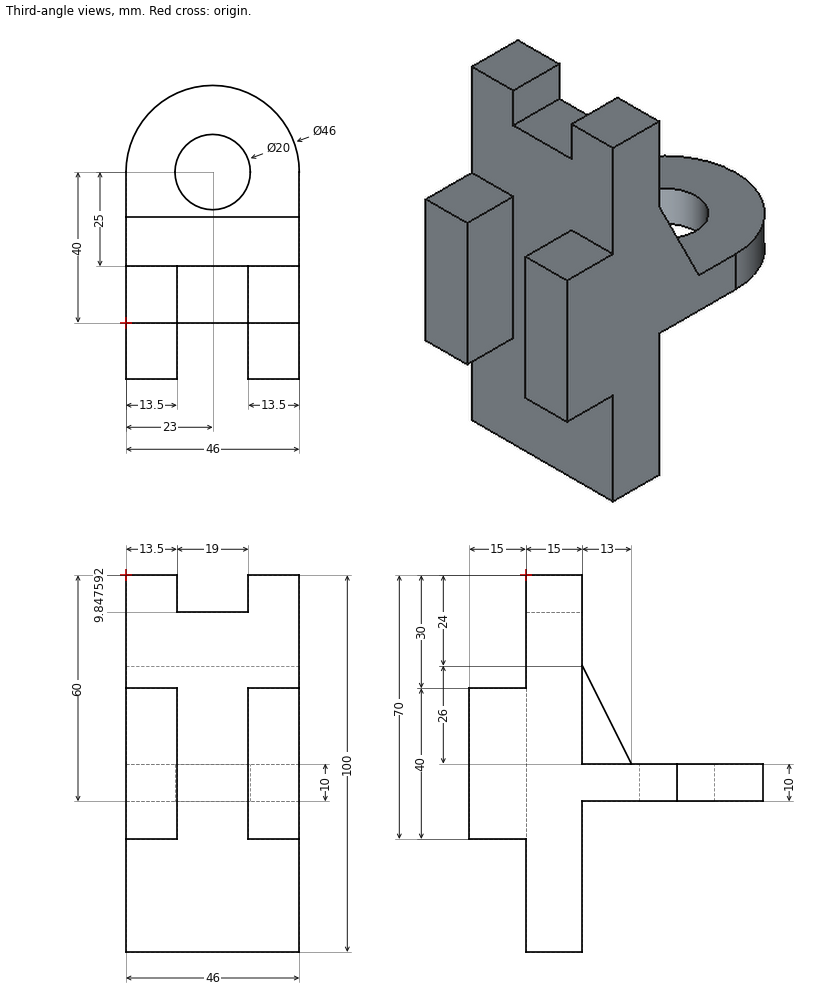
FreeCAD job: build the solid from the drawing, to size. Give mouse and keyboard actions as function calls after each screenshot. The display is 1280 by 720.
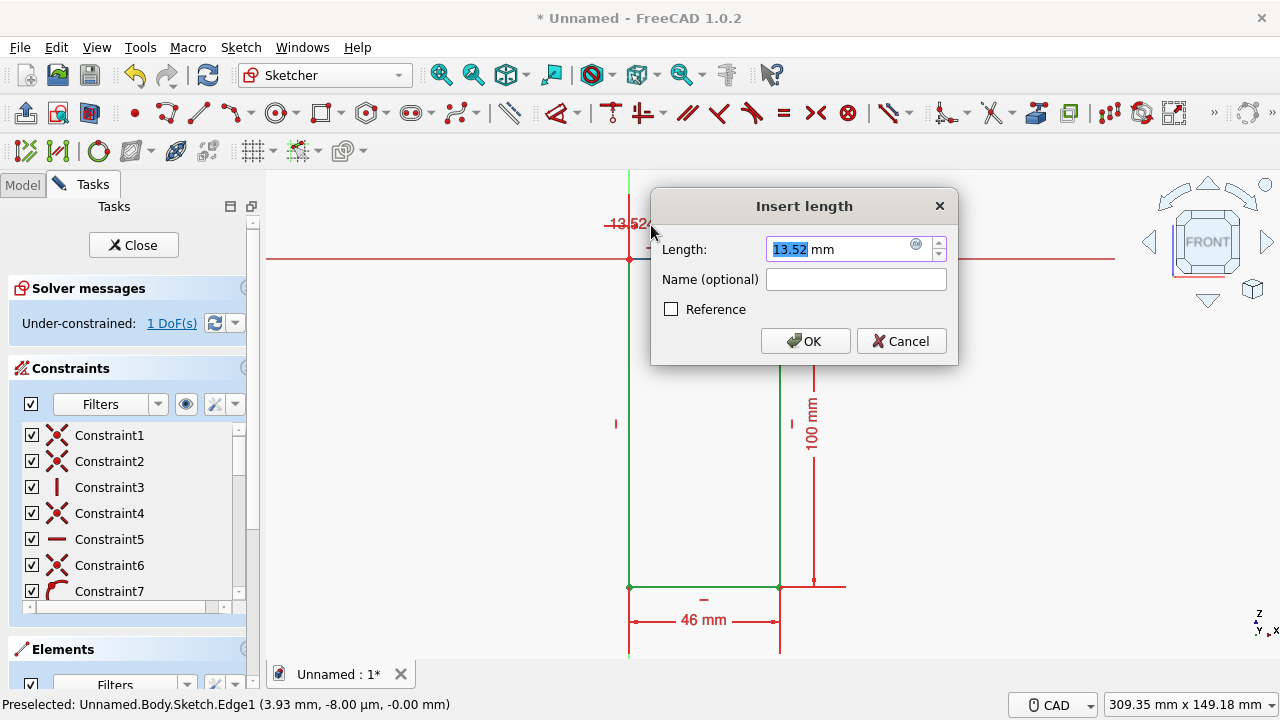
text(13.5)
key(Return)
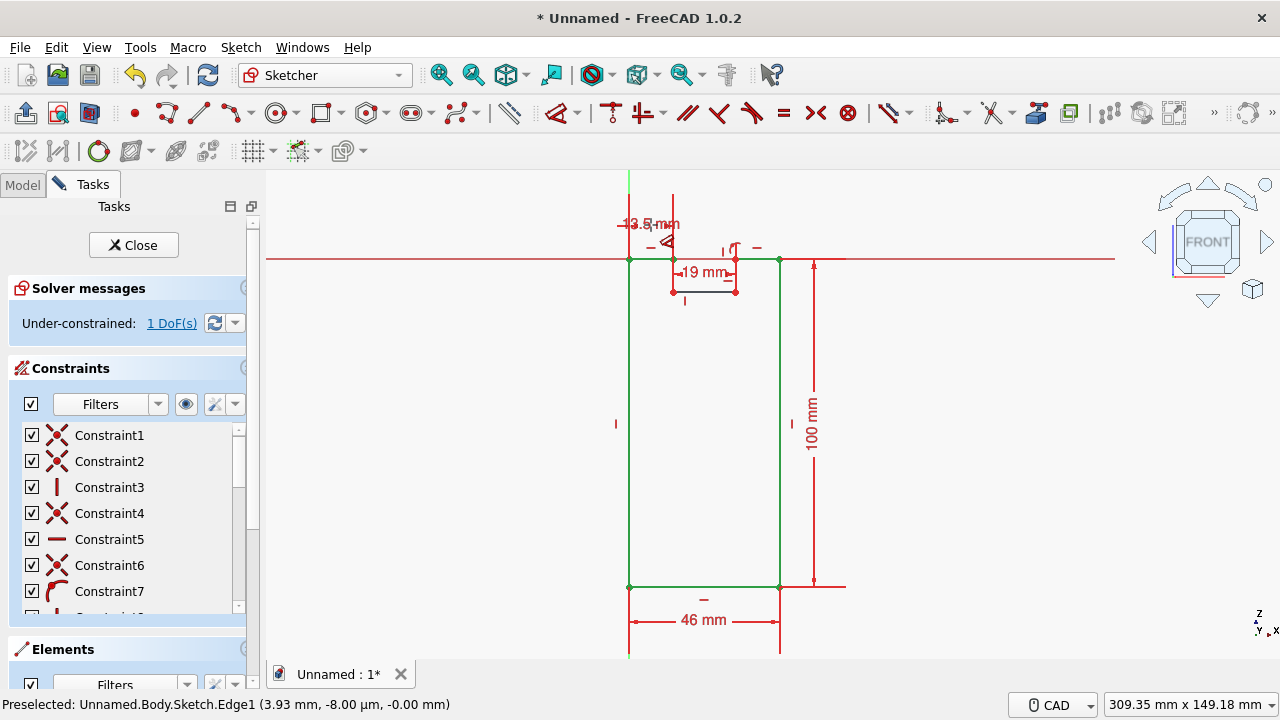
scroll(673, 269, up, 2)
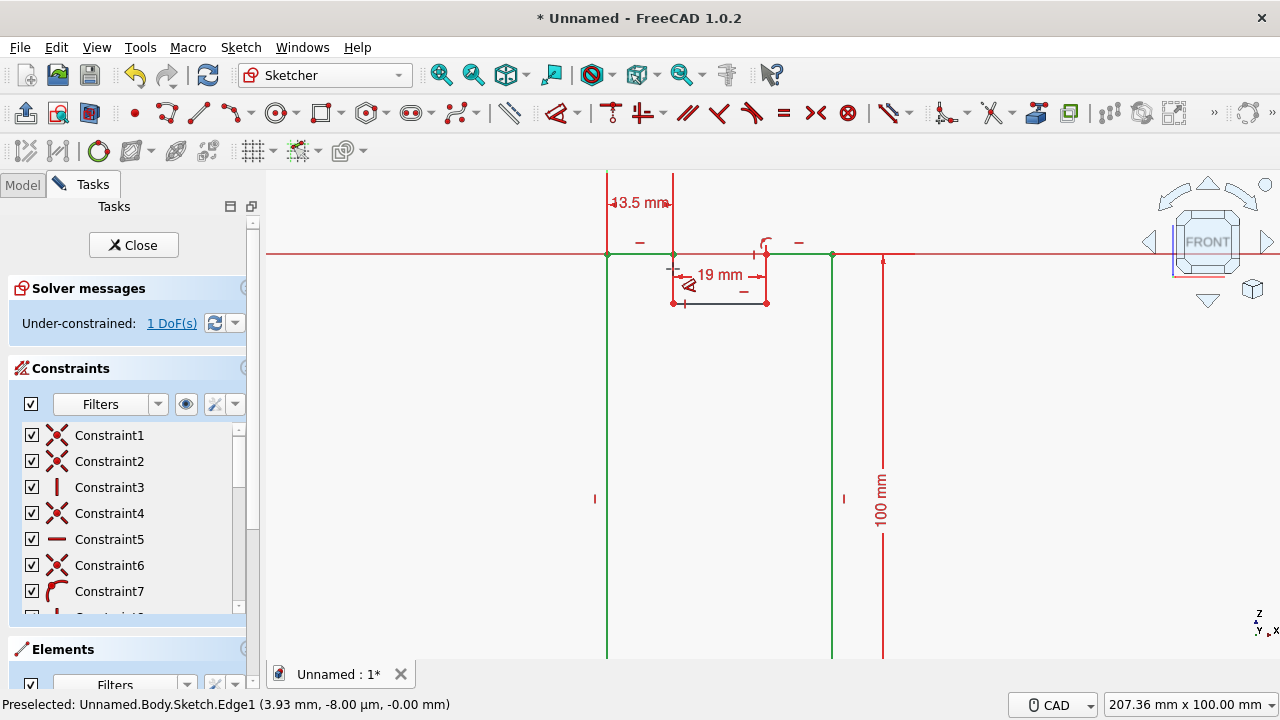
click(673, 269)
click(639, 279)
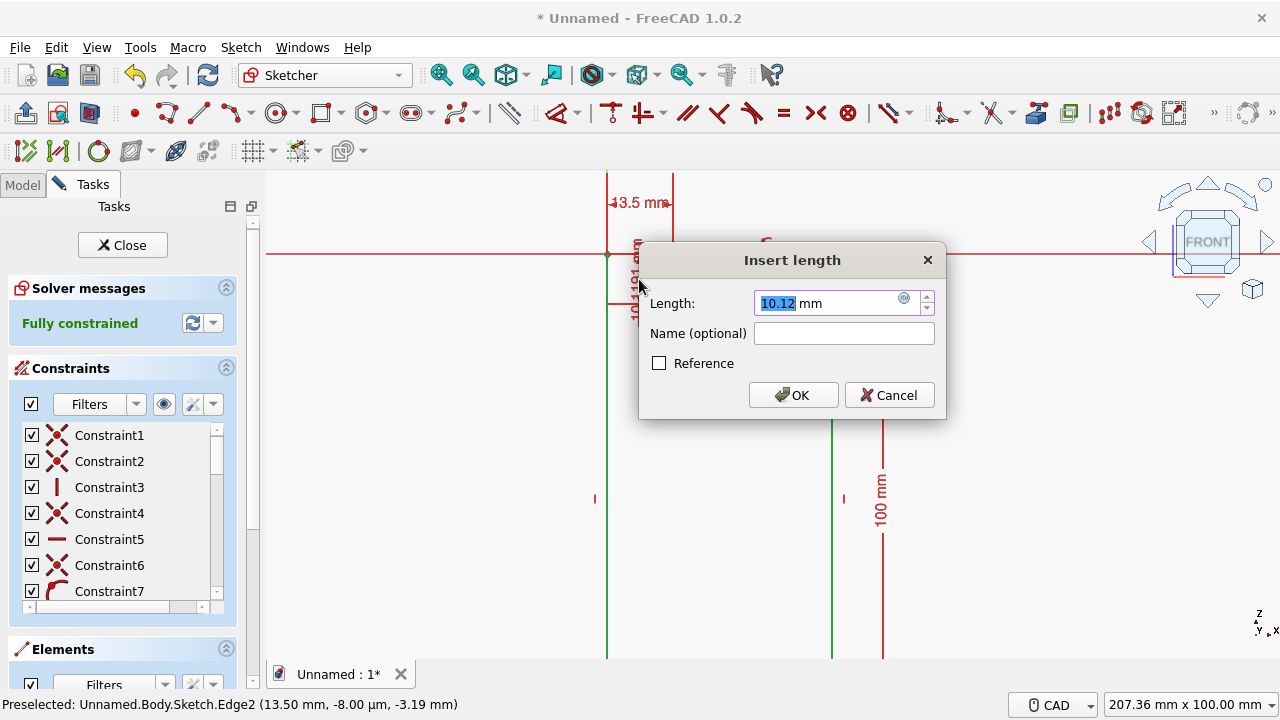
text(9.847592)
key(Return)
key(Escape)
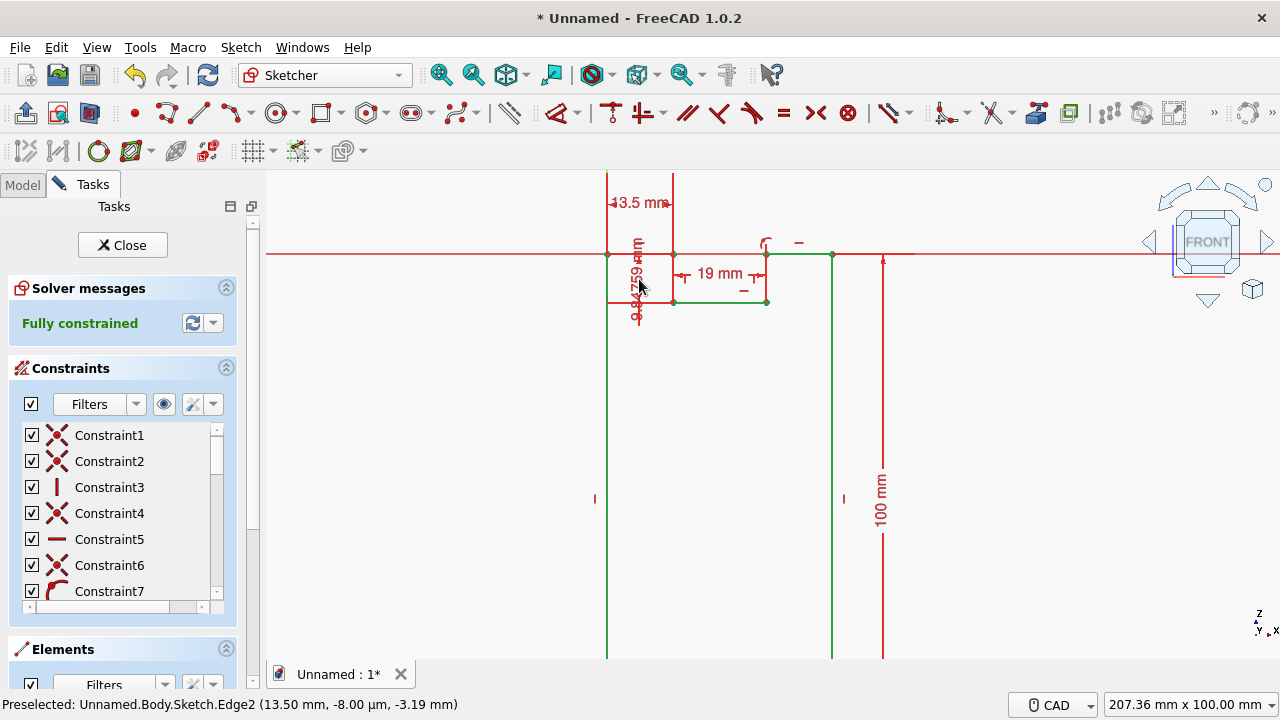
click(123, 245)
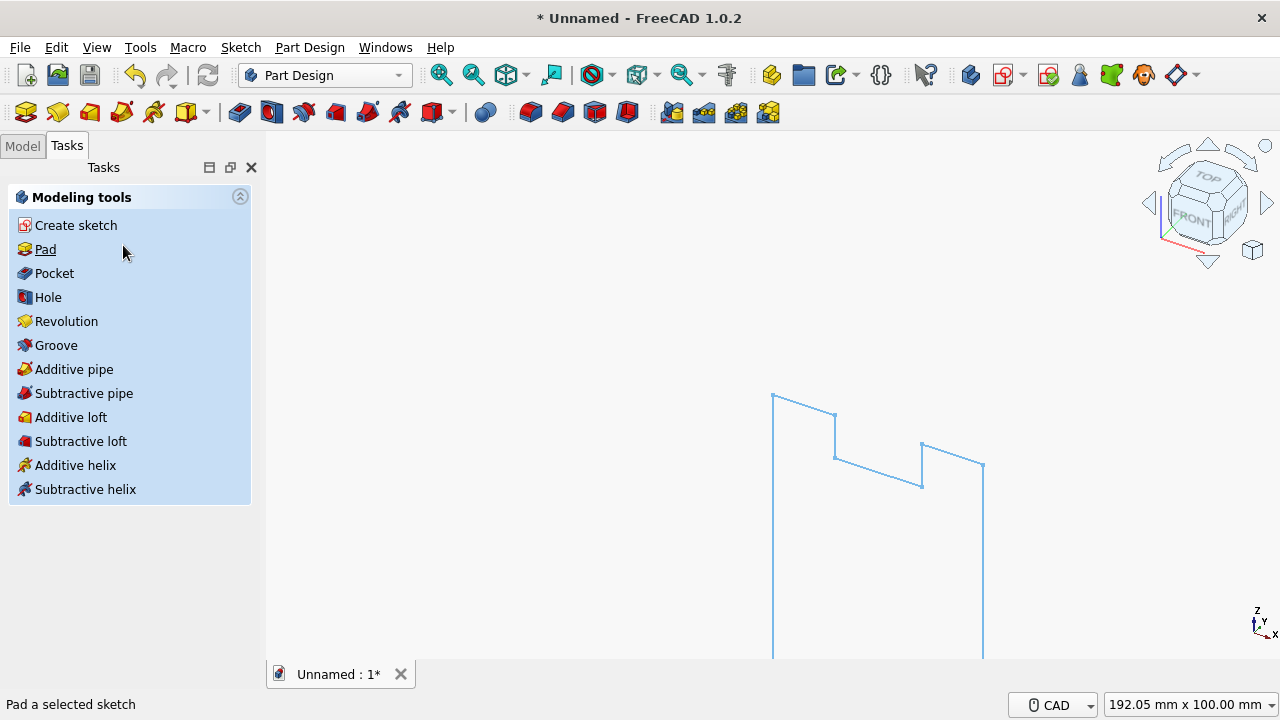
click(26, 112)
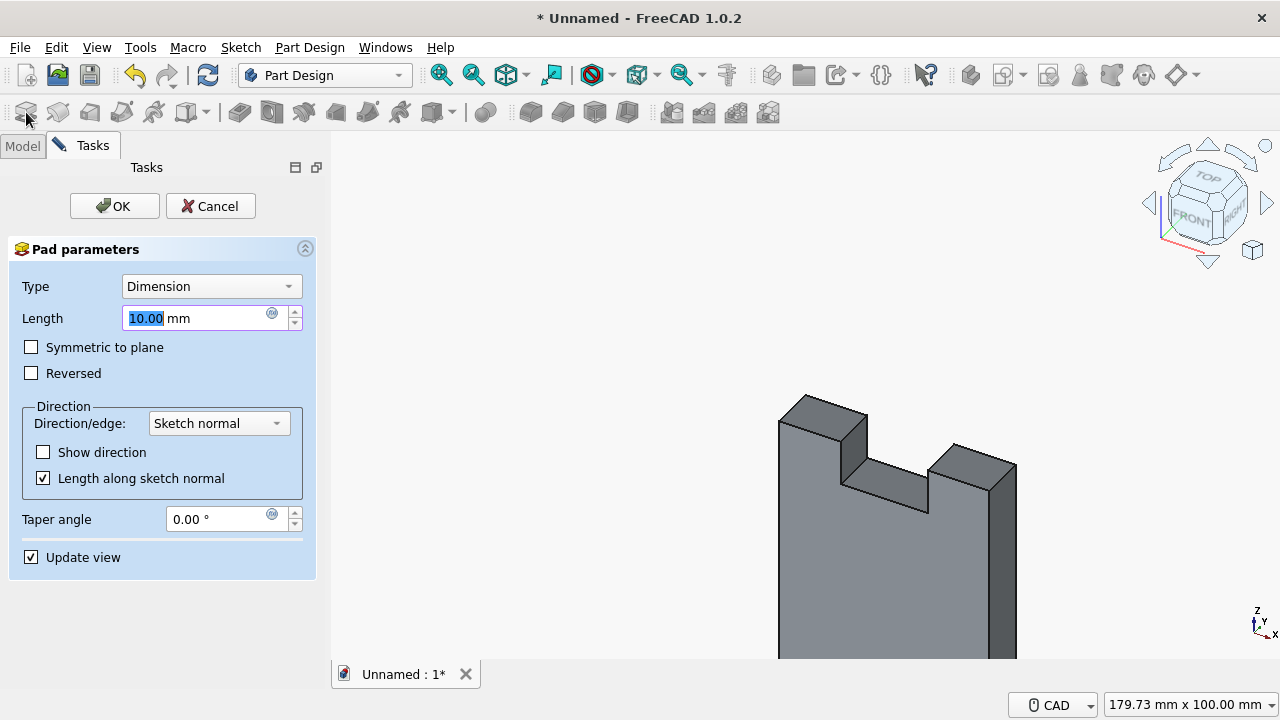
text(15)
key(Tab)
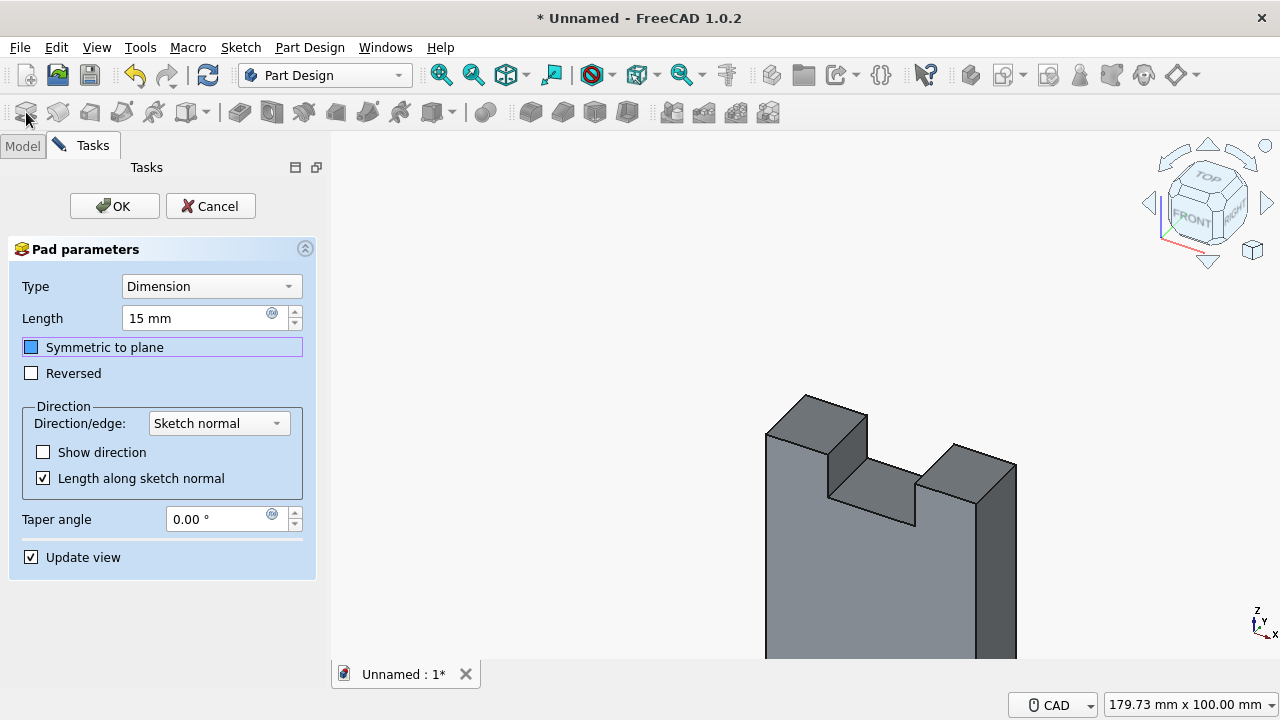
click(30, 373)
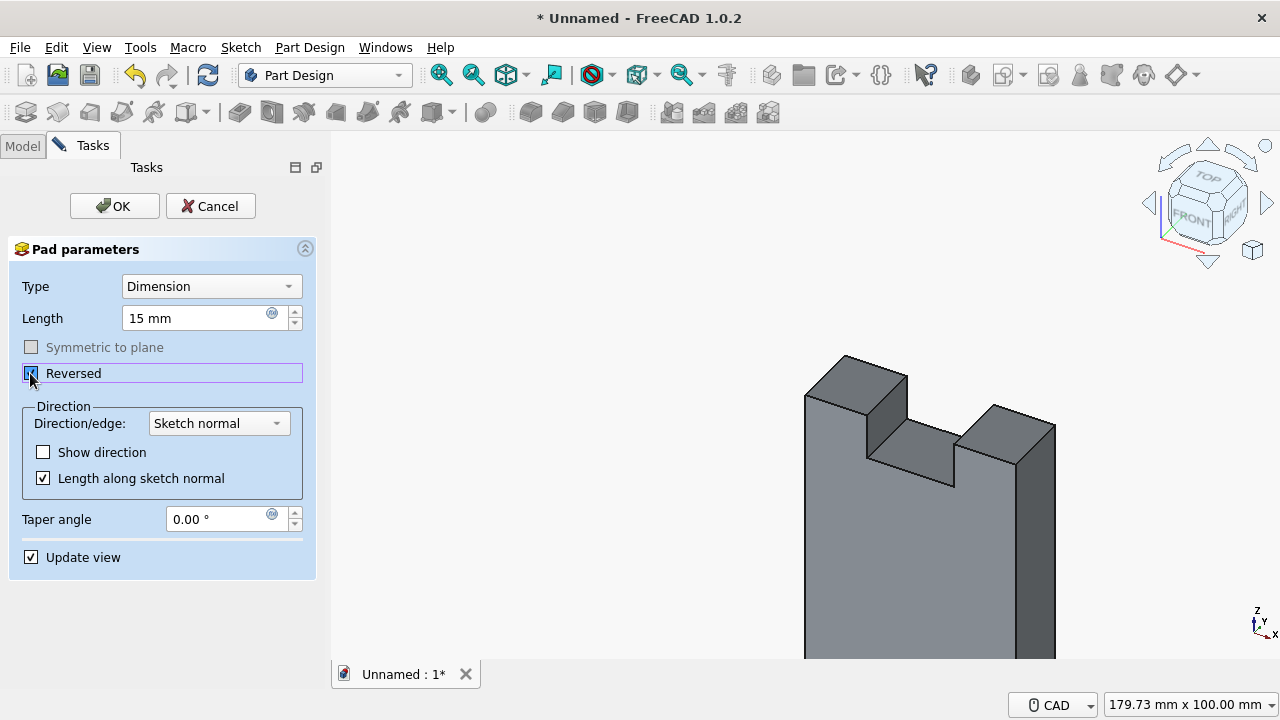
click(115, 206)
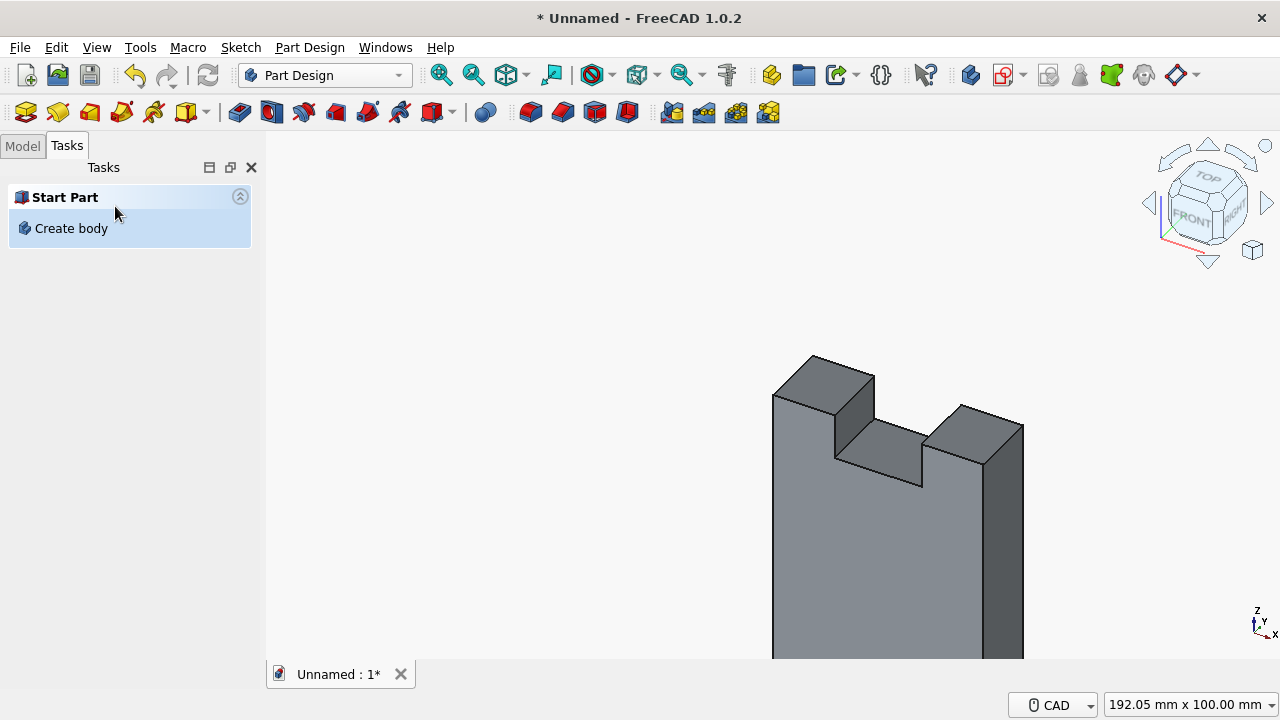
key(v)
key(f)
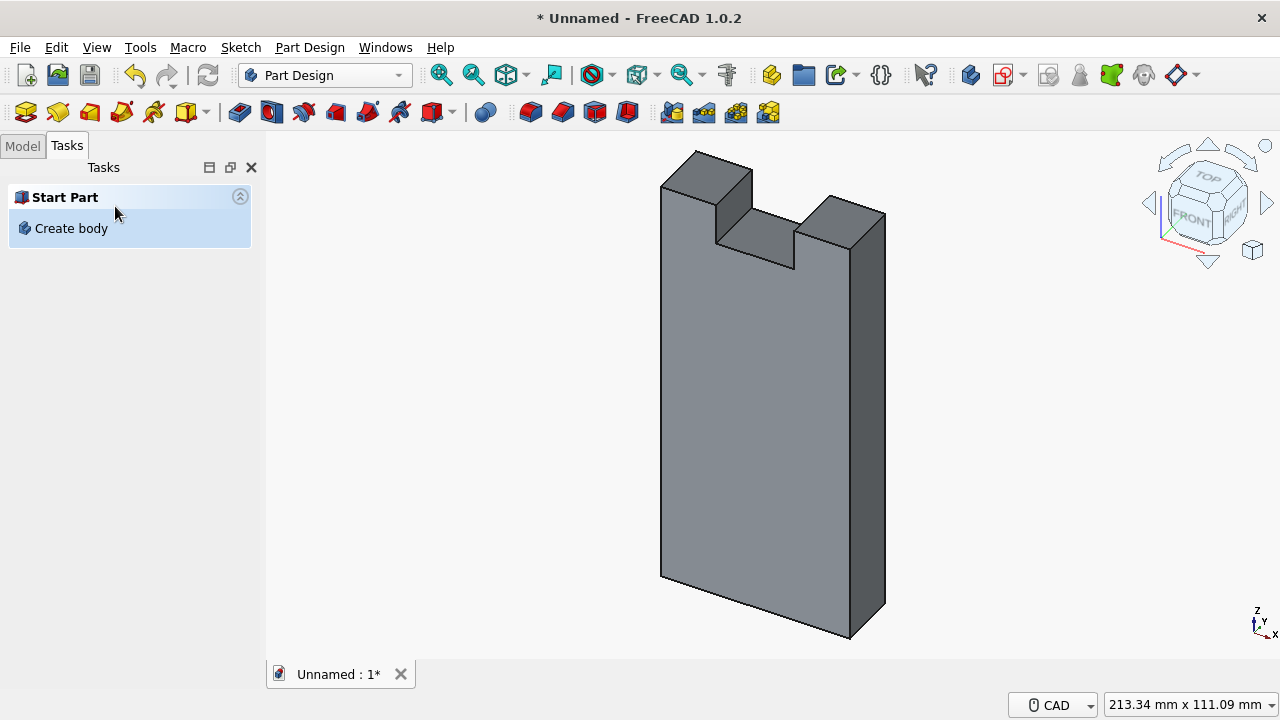
key(6)